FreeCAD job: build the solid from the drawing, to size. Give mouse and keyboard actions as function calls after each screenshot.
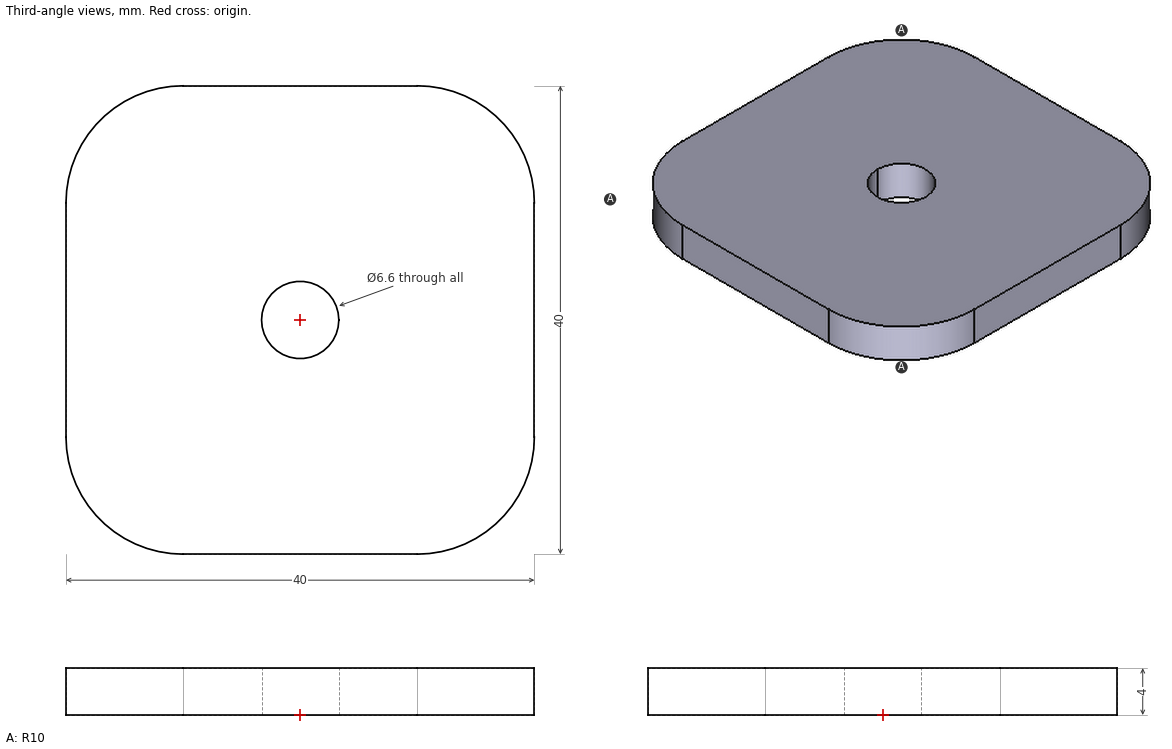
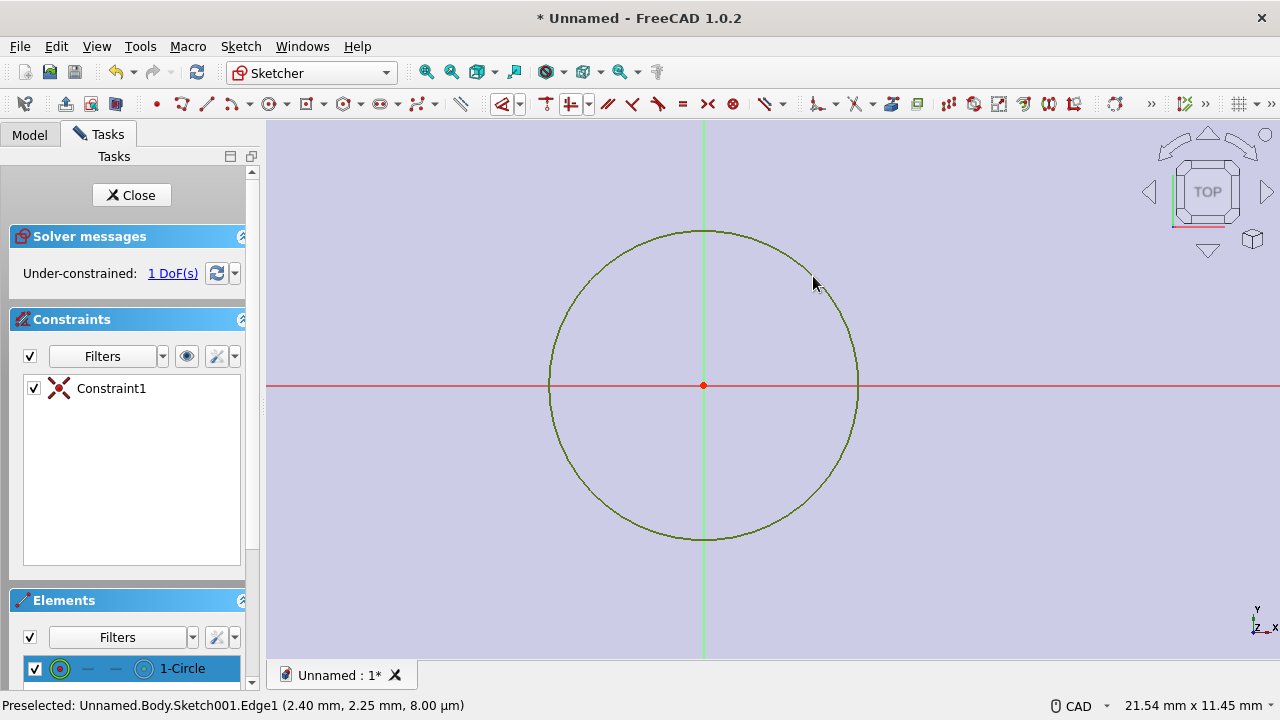
key(k)
key(o)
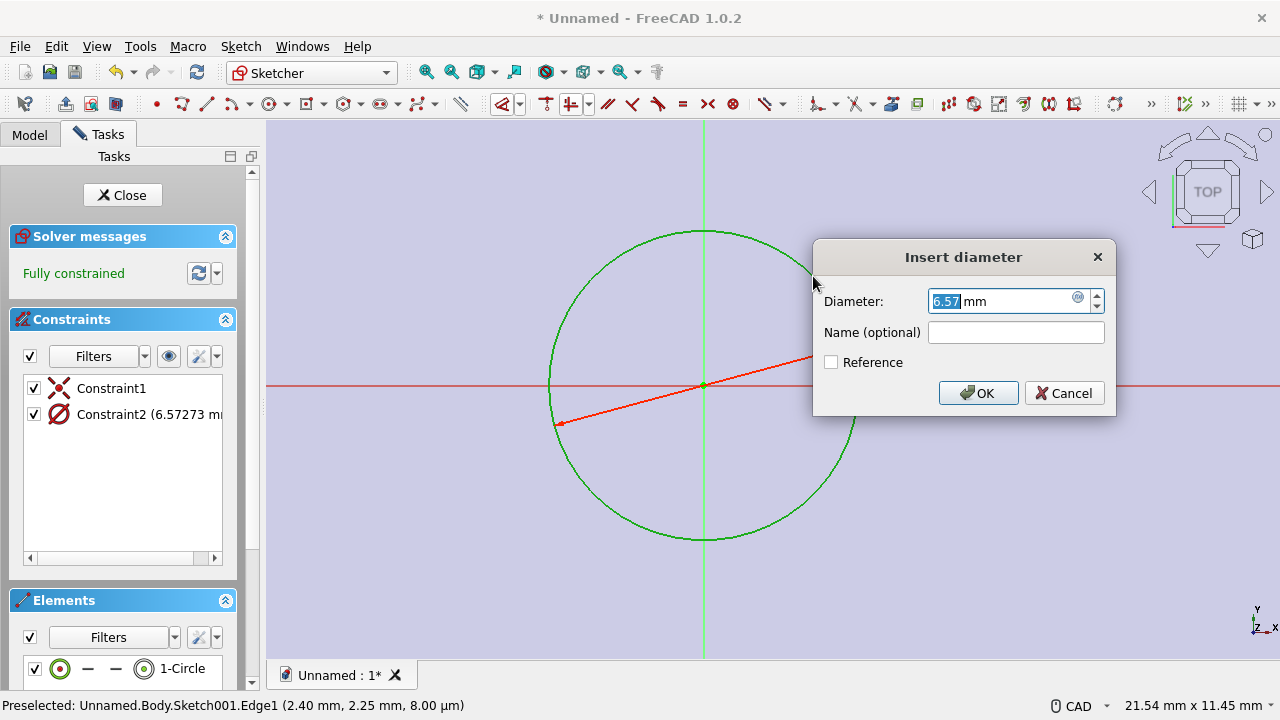
text(6.6)
key(Return)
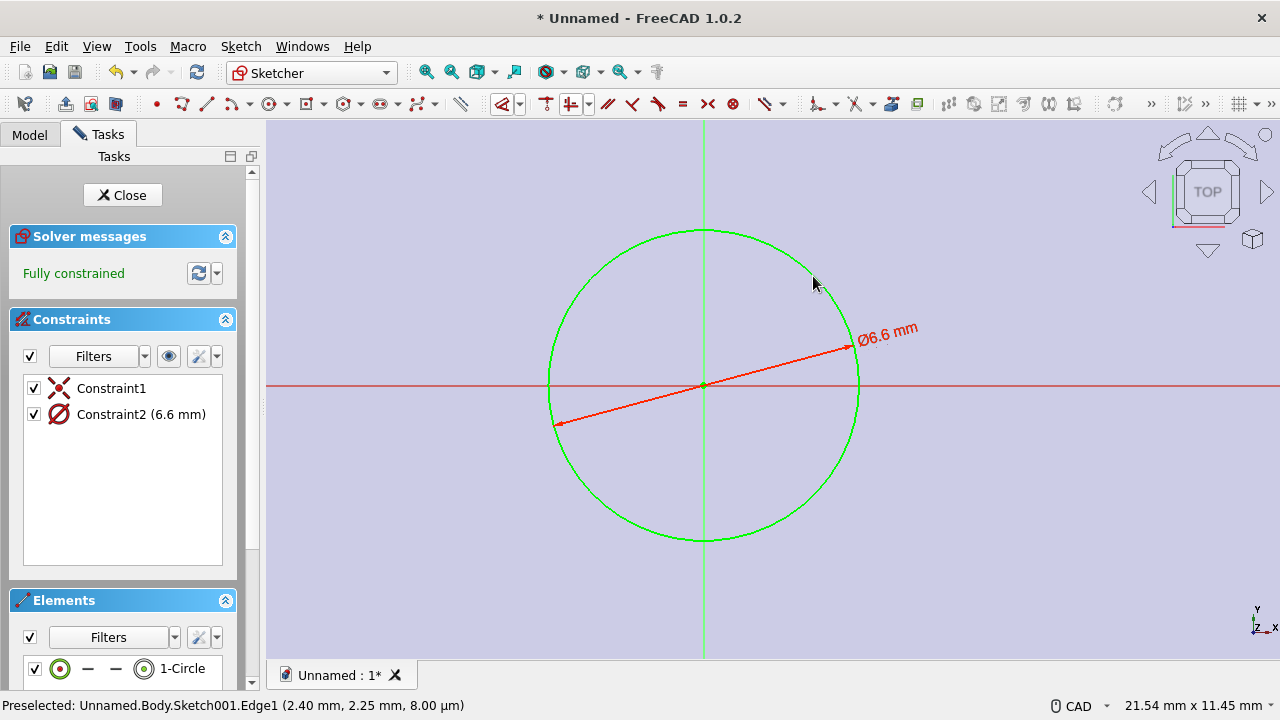
click(123, 195)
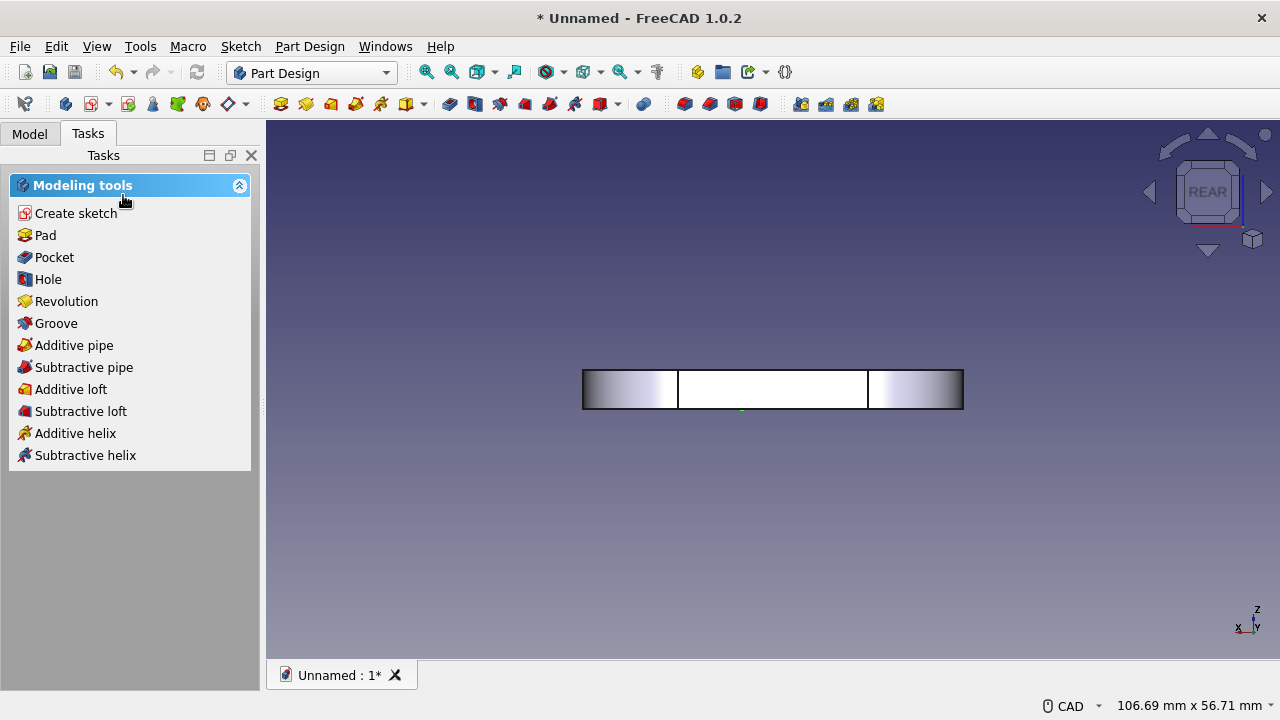
click(475, 104)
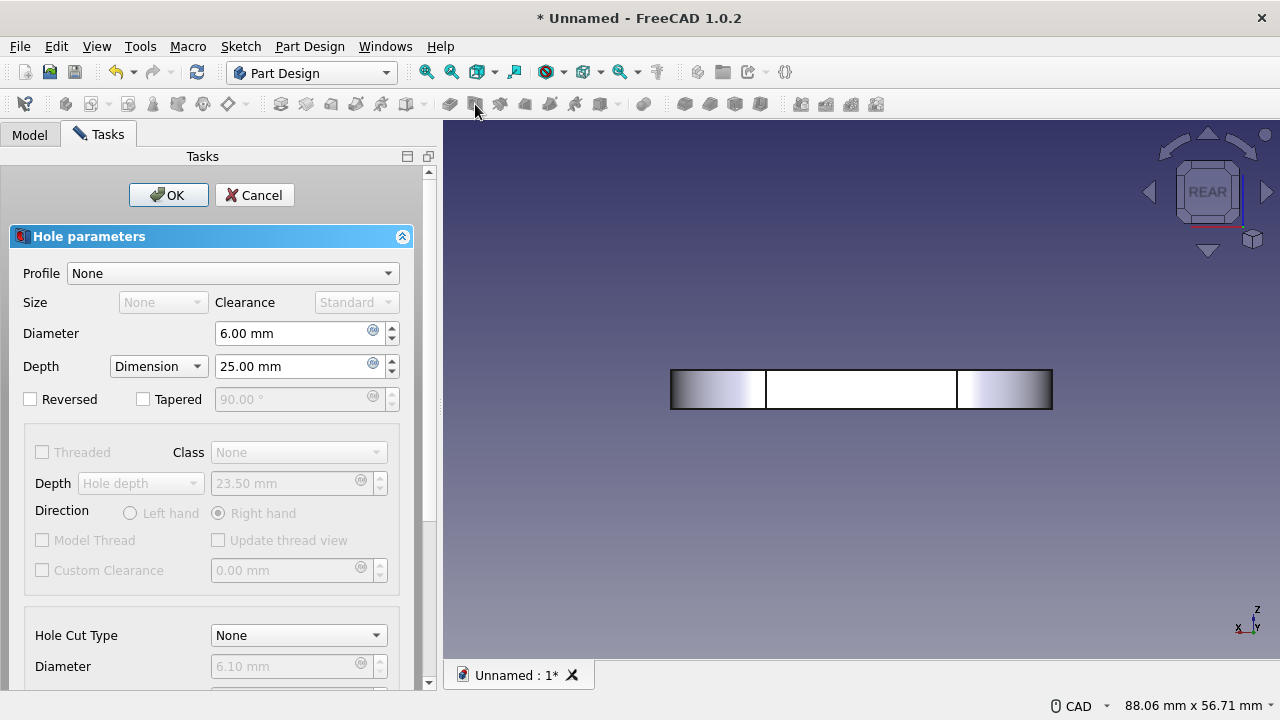
triple_click(300, 334)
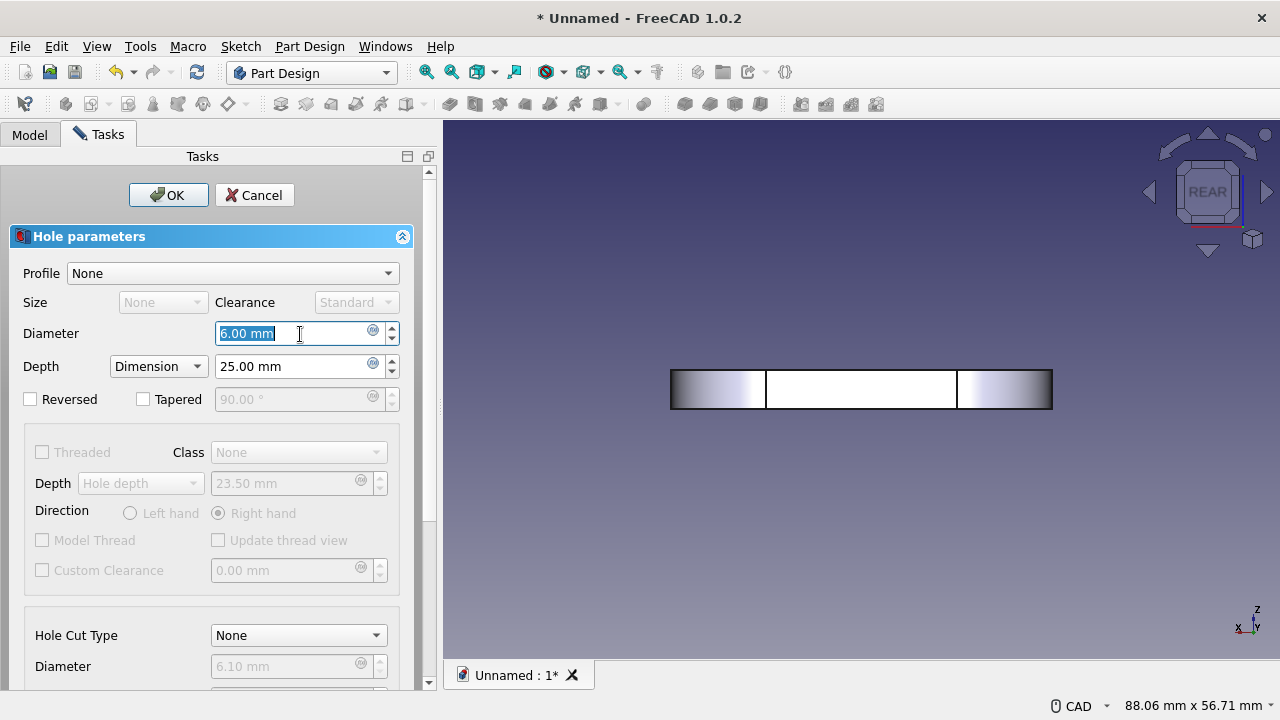
text(6.6)
key(Tab)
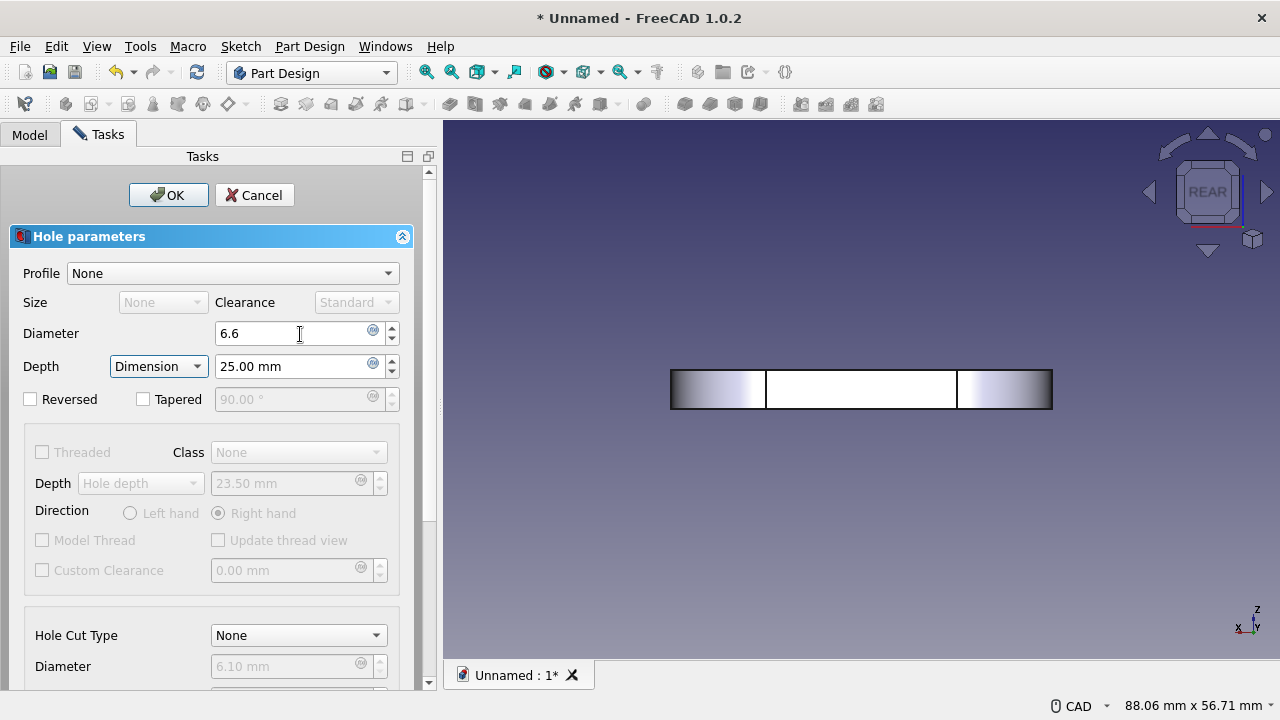
click(160, 366)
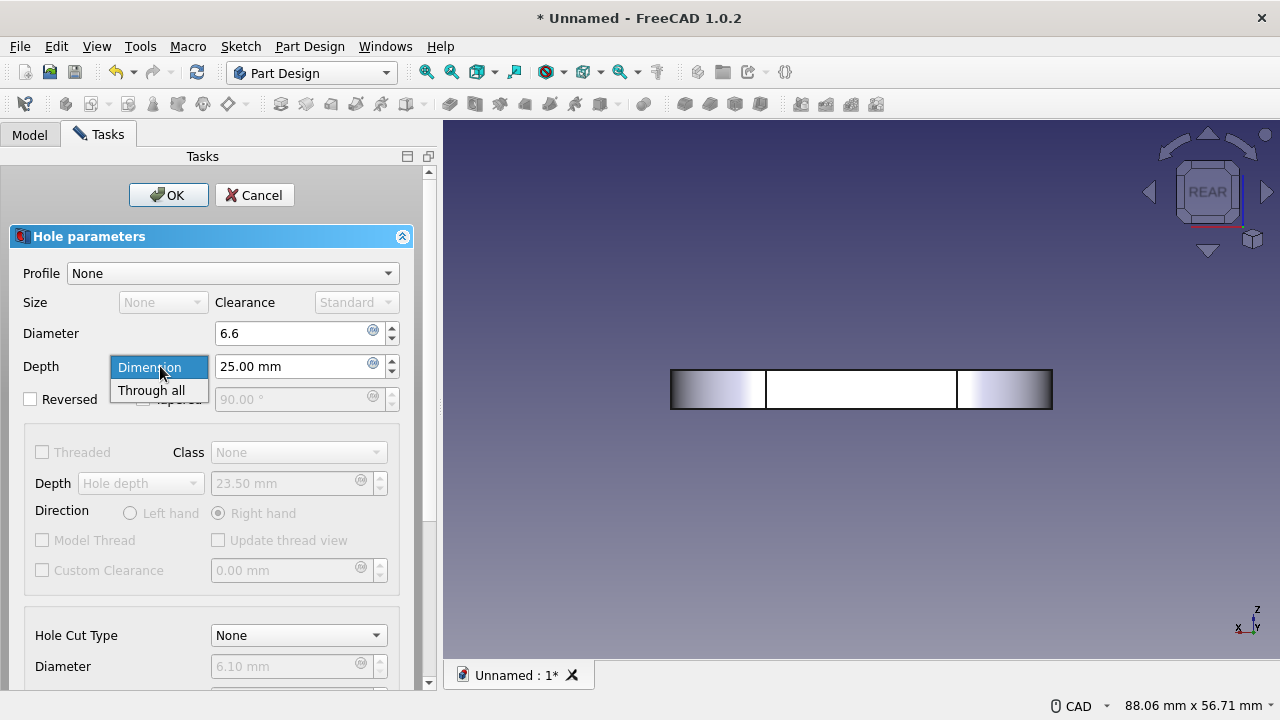
click(158, 390)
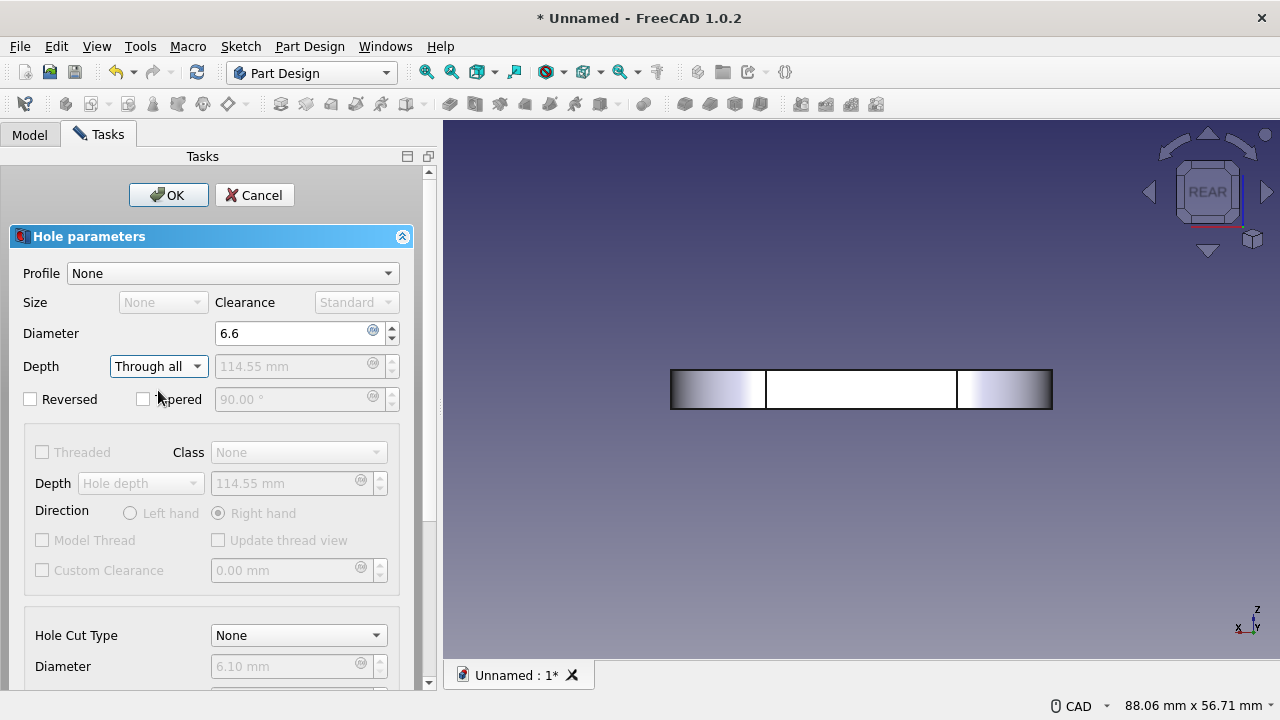
click(31, 399)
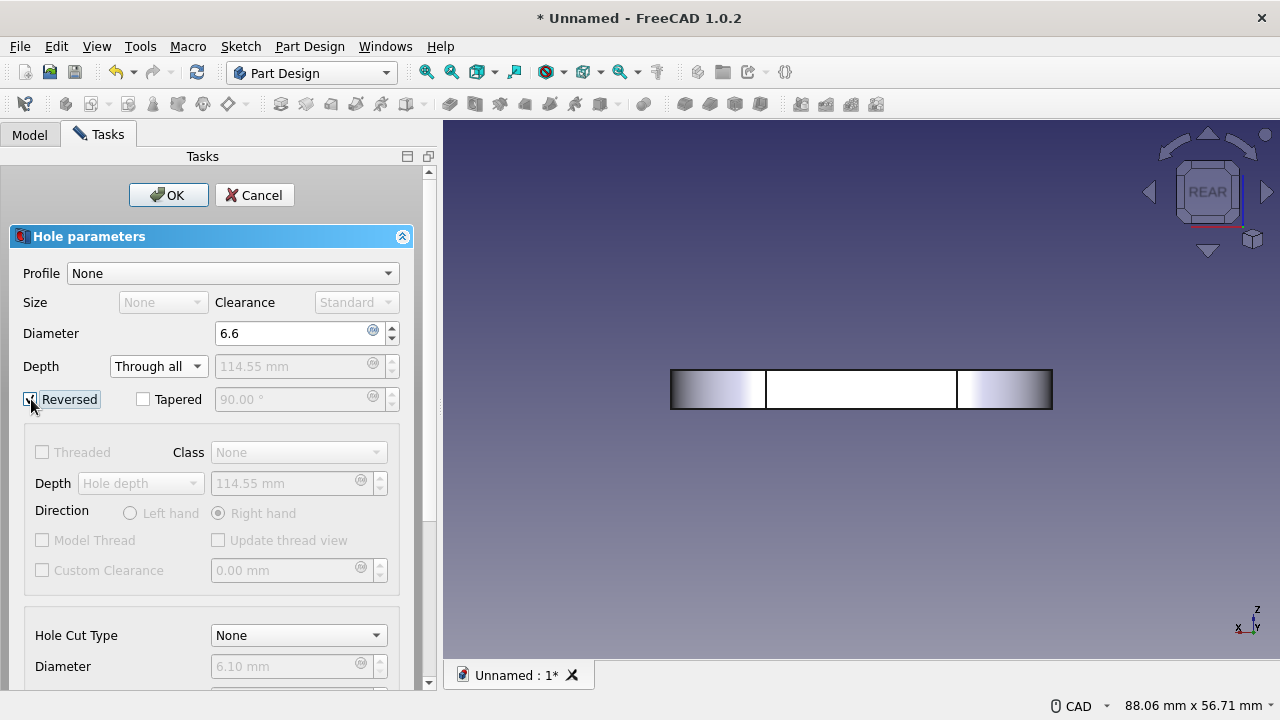
click(169, 195)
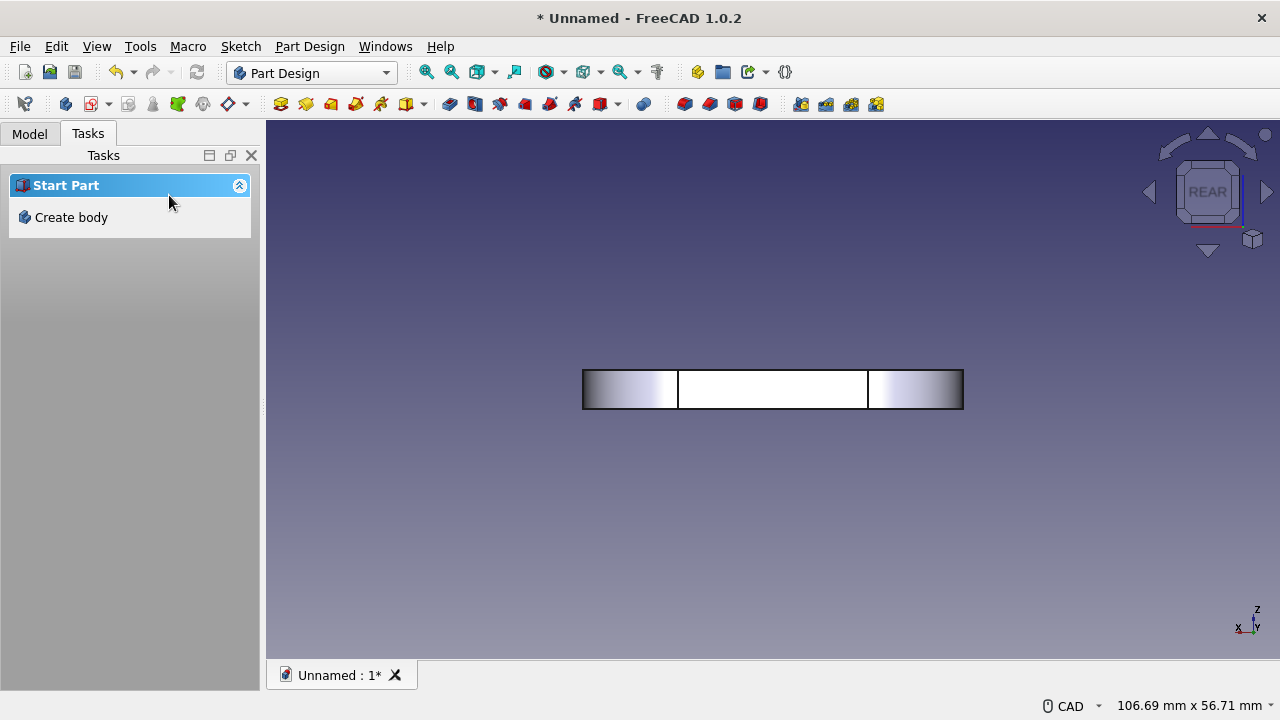
key(0)